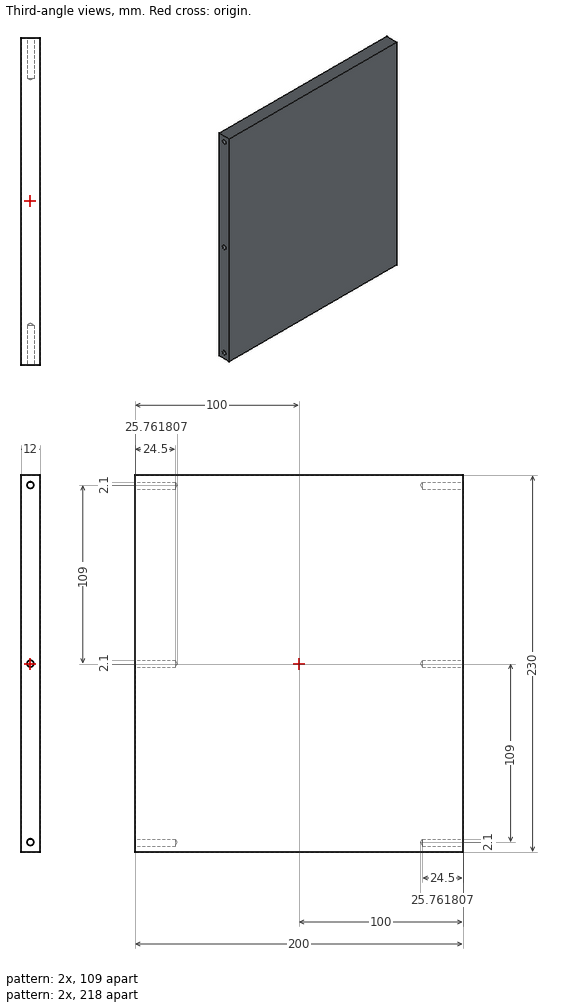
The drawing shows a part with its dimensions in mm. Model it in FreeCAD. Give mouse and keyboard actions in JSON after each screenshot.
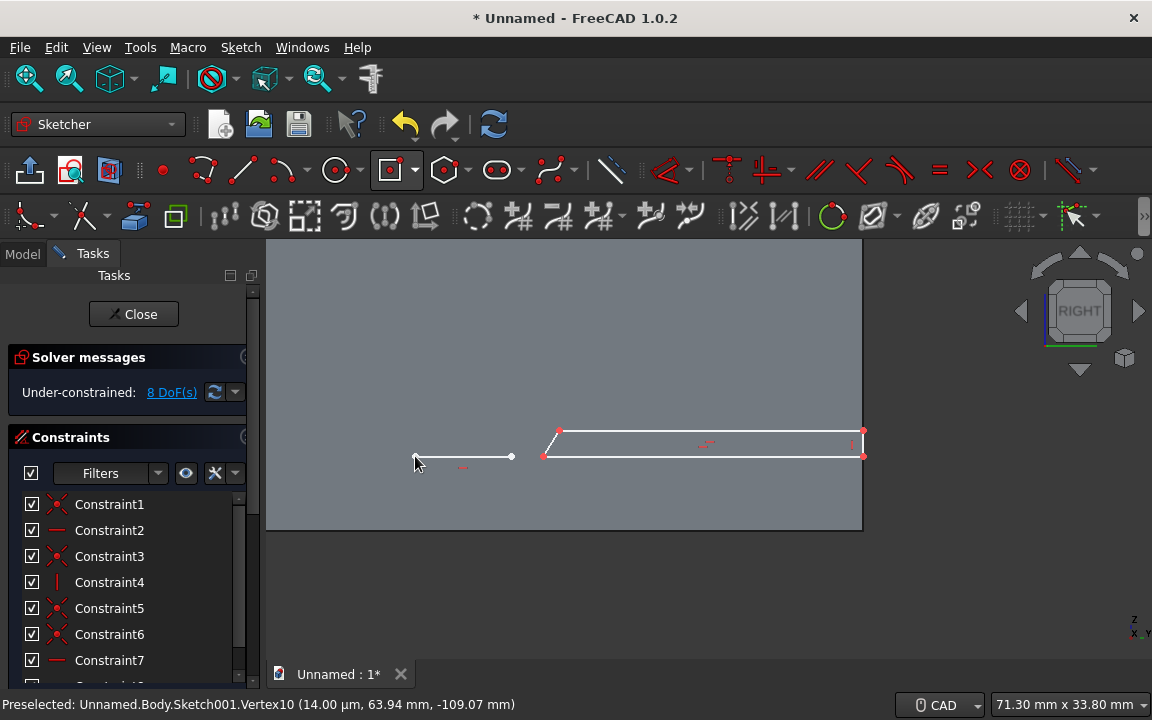
{"action": "left_click", "coordinate": [482, 457]}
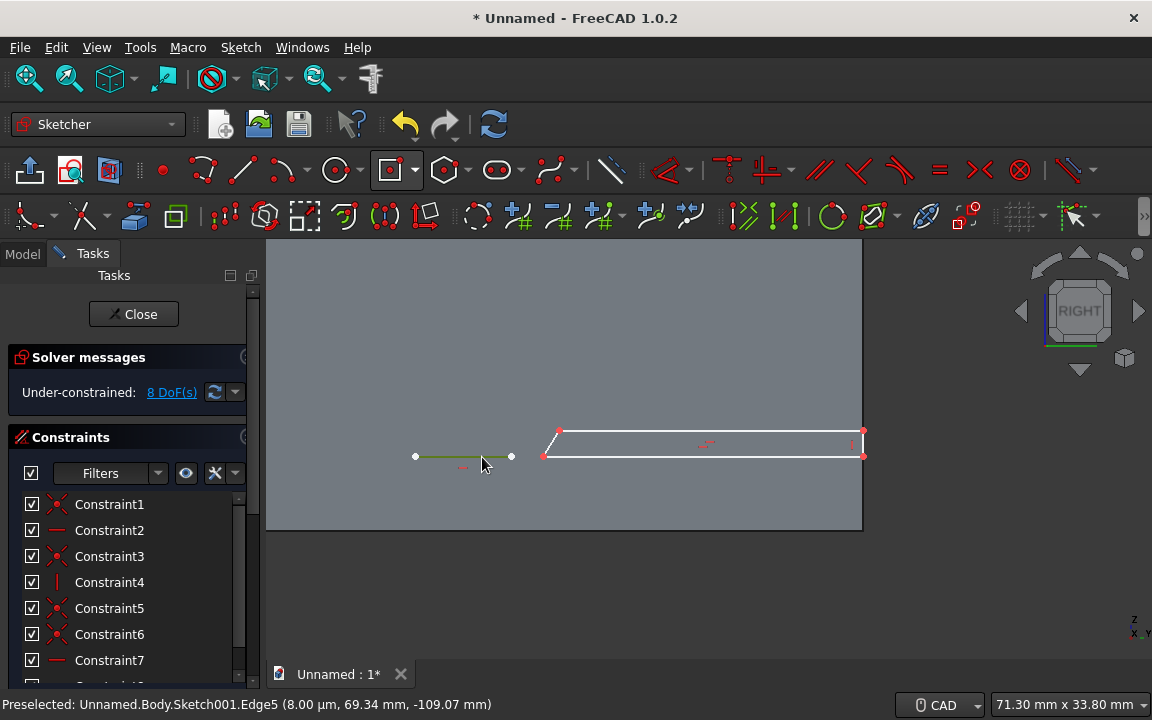
{"action": "left_click", "coordinate": [612, 170]}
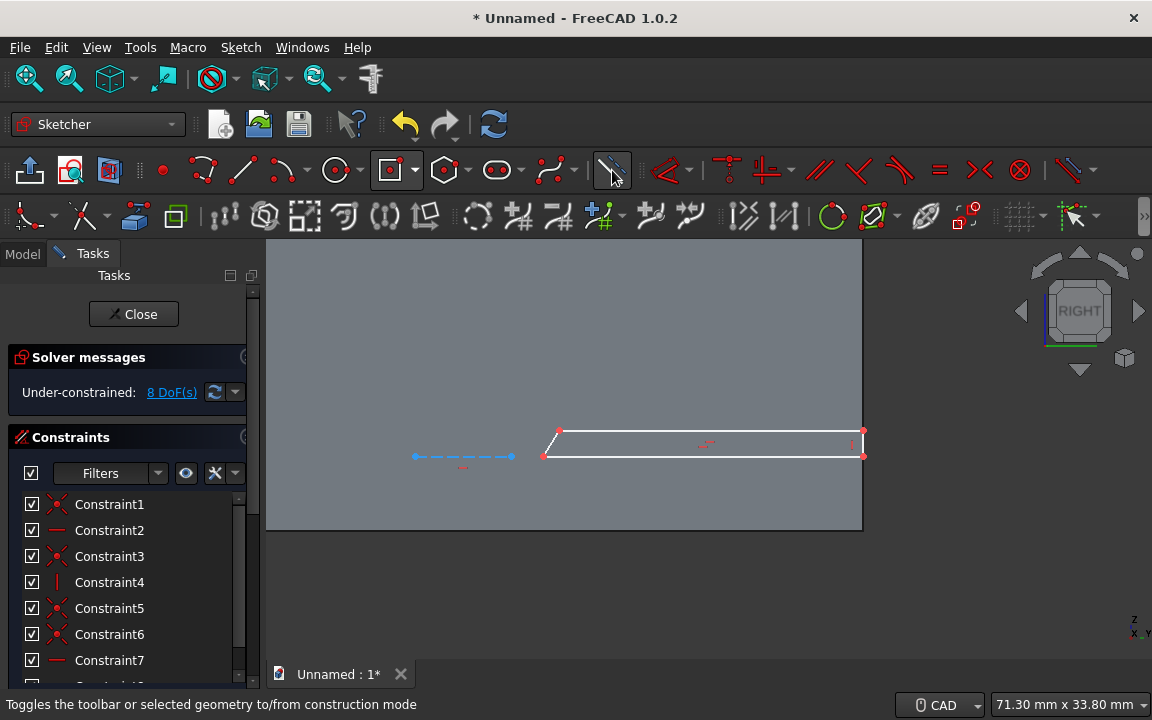
{"action": "left_click", "coordinate": [666, 170]}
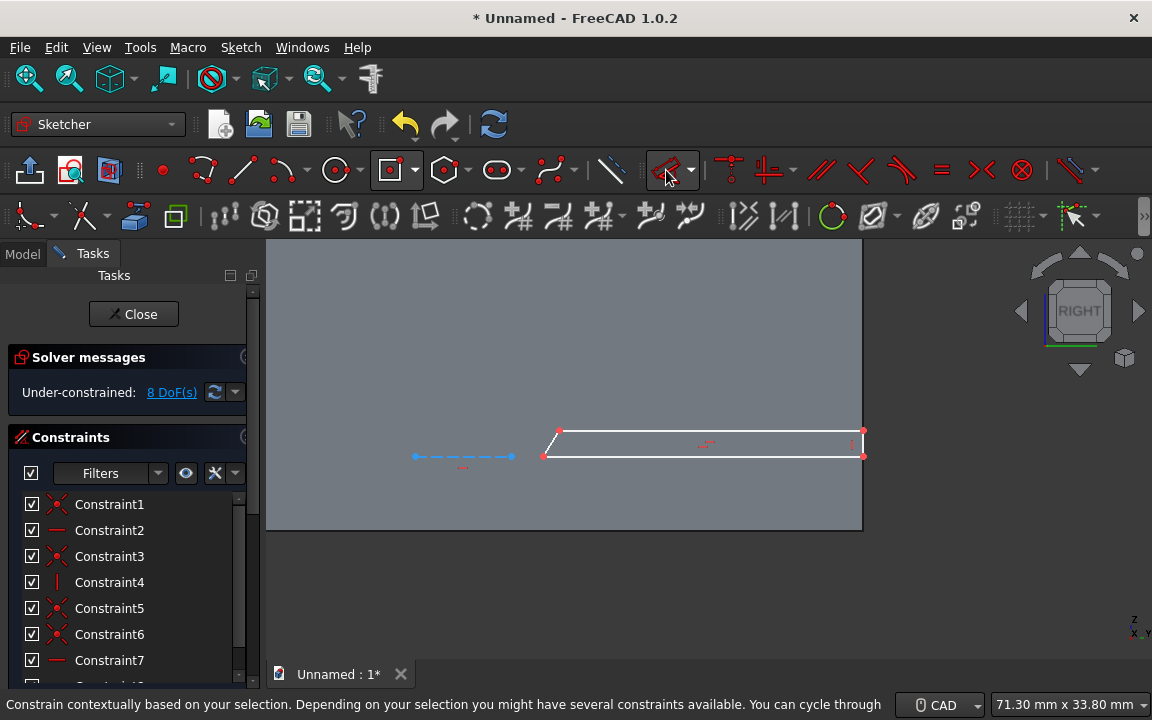
{"action": "scroll", "coordinate": [863, 447], "scroll_direction": "up", "scroll_amount": 3}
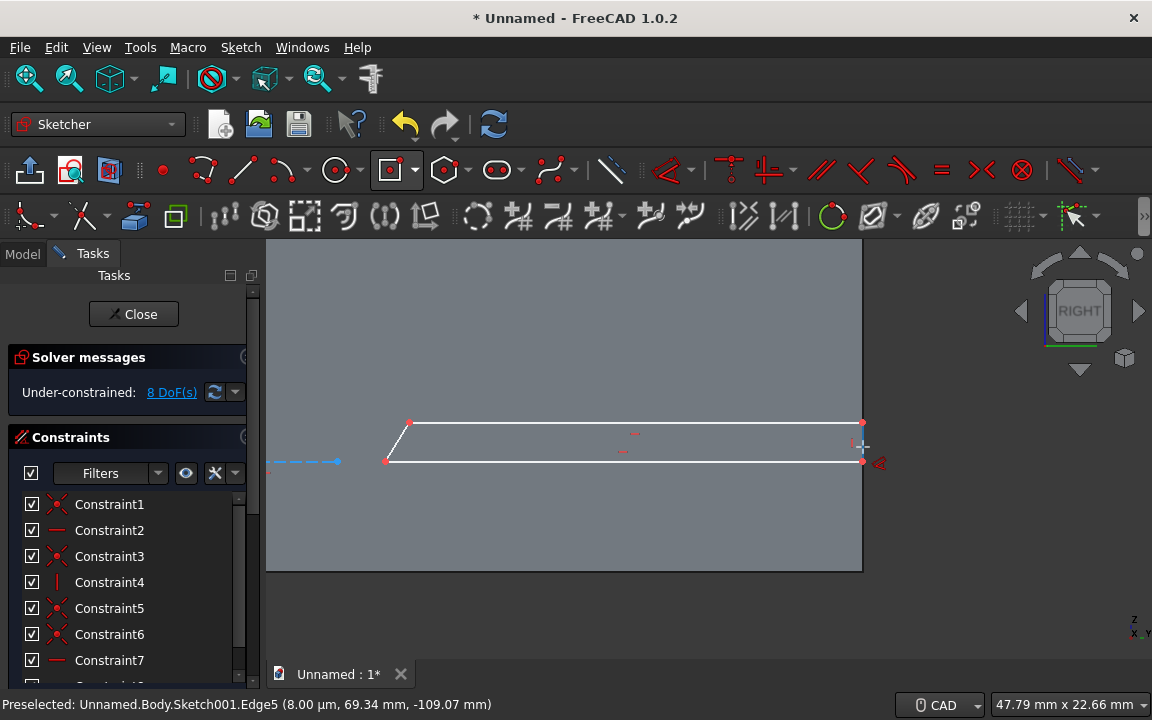
{"action": "left_click", "coordinate": [862, 446]}
{"action": "left_click", "coordinate": [896, 441]}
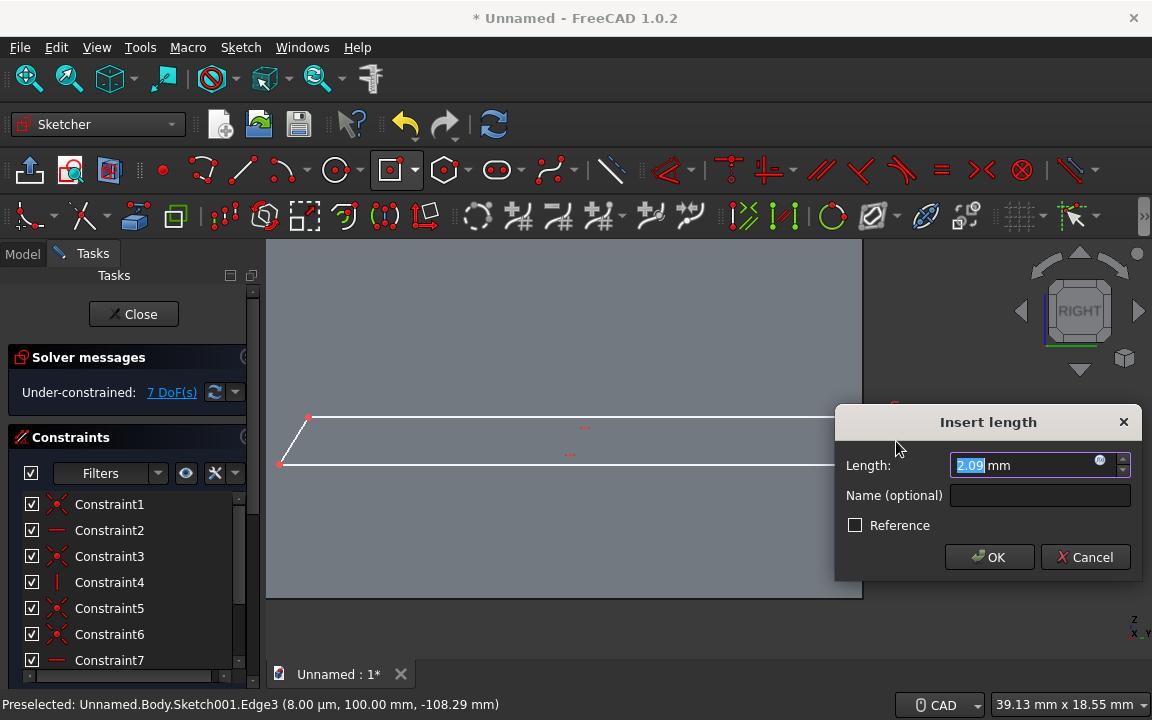
{"action": "type", "text": "2.1"}
{"action": "key", "text": "Return"}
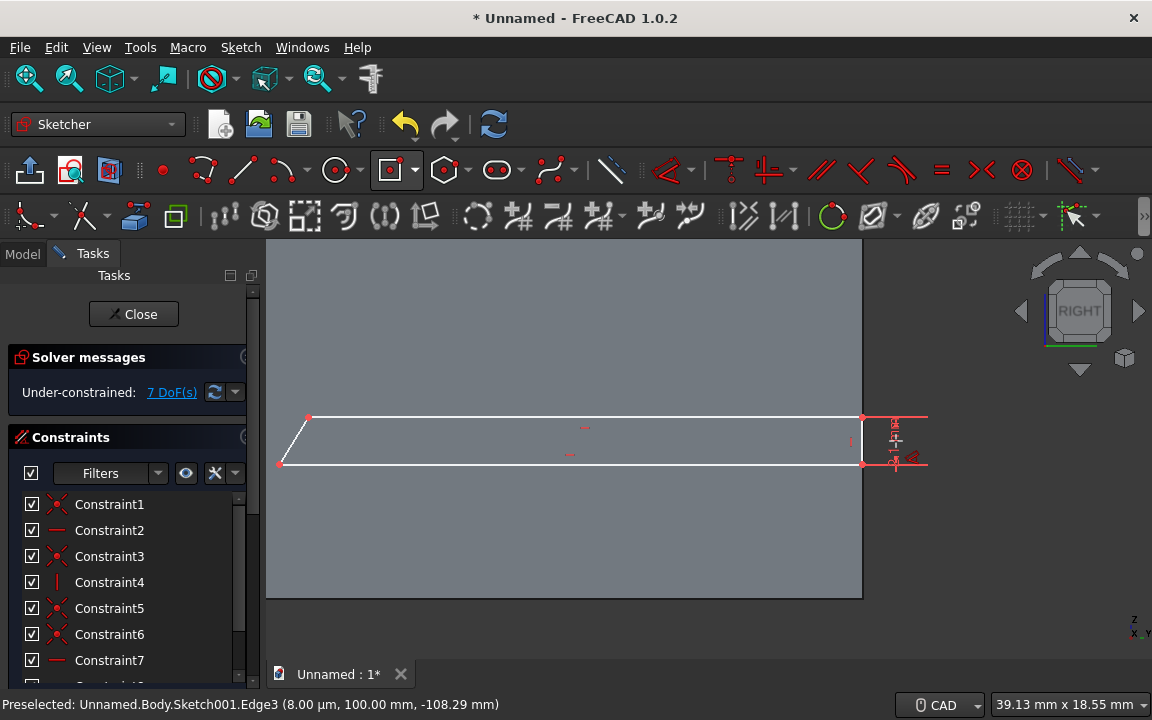
{"action": "left_click", "coordinate": [696, 417]}
{"action": "left_click", "coordinate": [585, 383]}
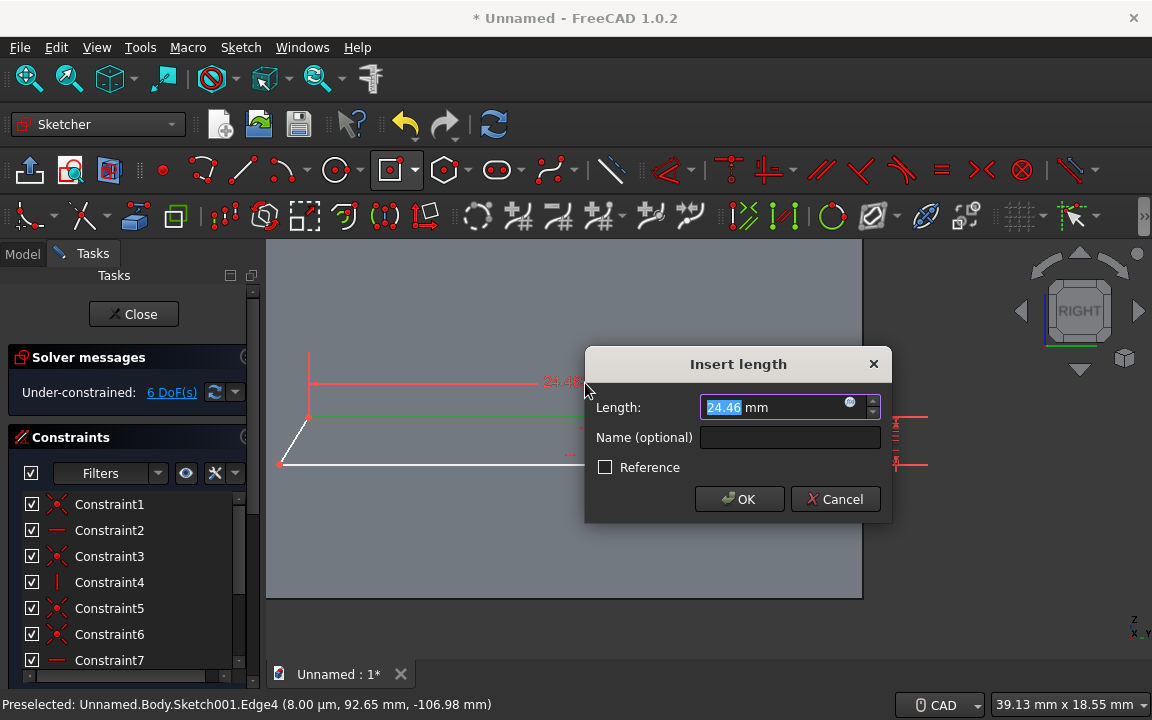
{"action": "type", "text": "24.5"}
{"action": "key", "text": "Return"}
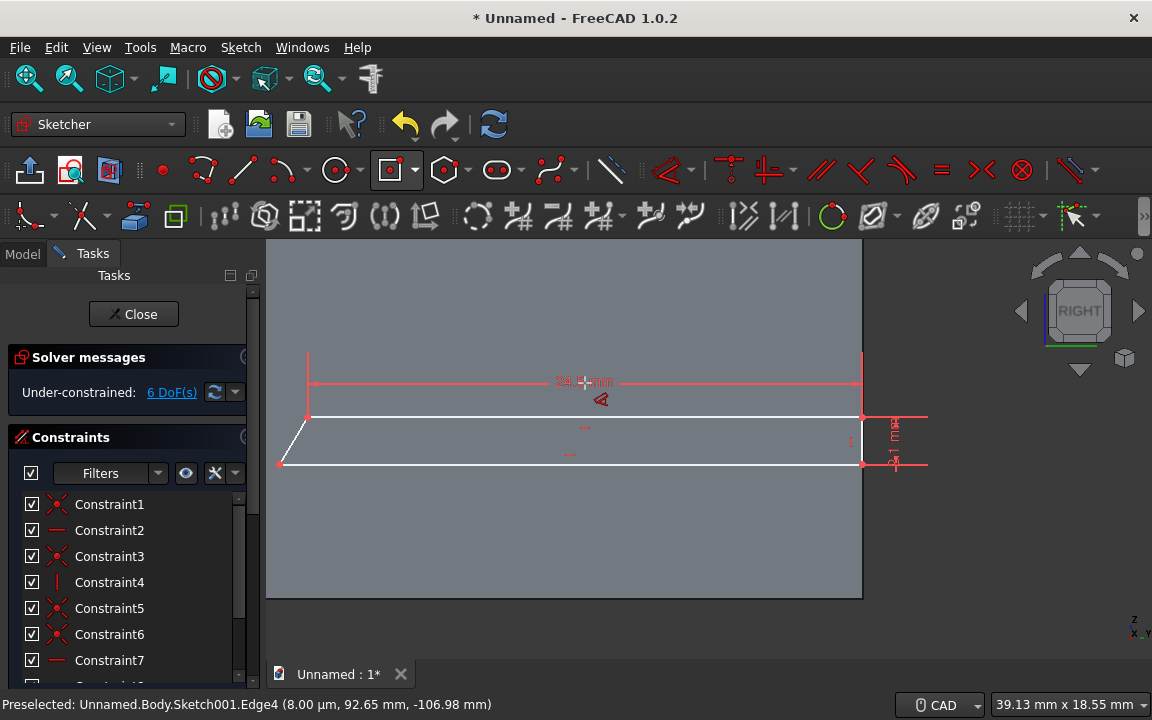
{"action": "scroll", "coordinate": [867, 461], "scroll_direction": "down", "scroll_amount": 3}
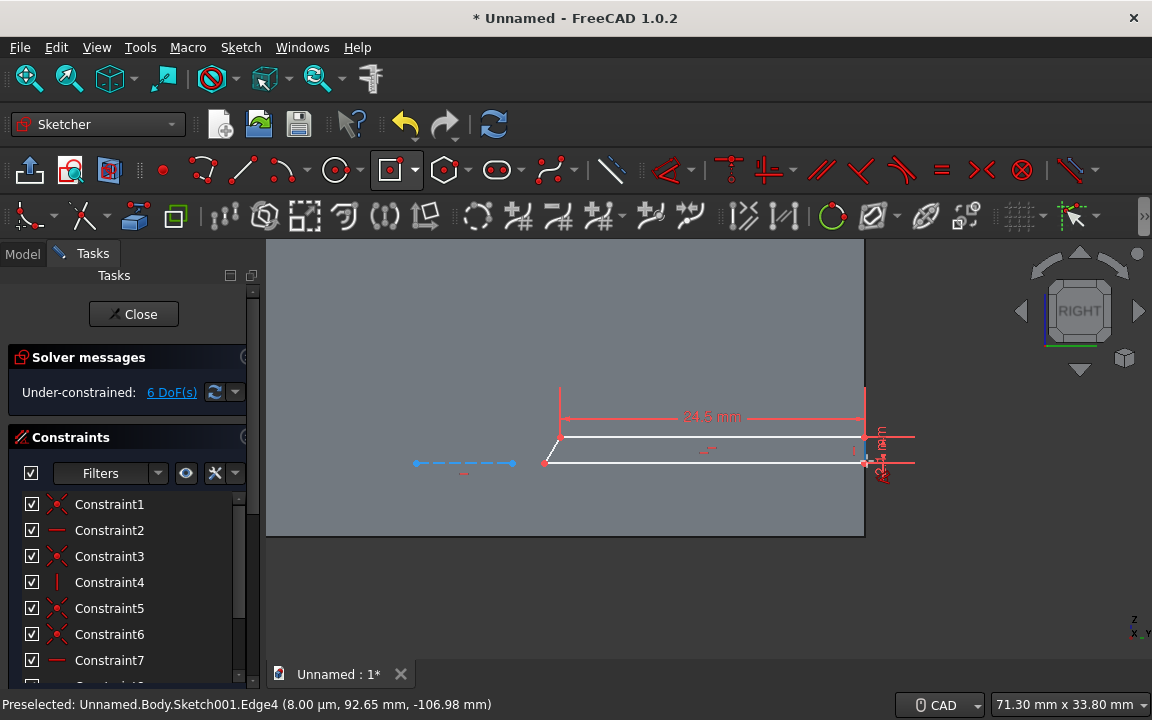
{"action": "left_click", "coordinate": [545, 463]}
{"action": "left_click", "coordinate": [579, 365]}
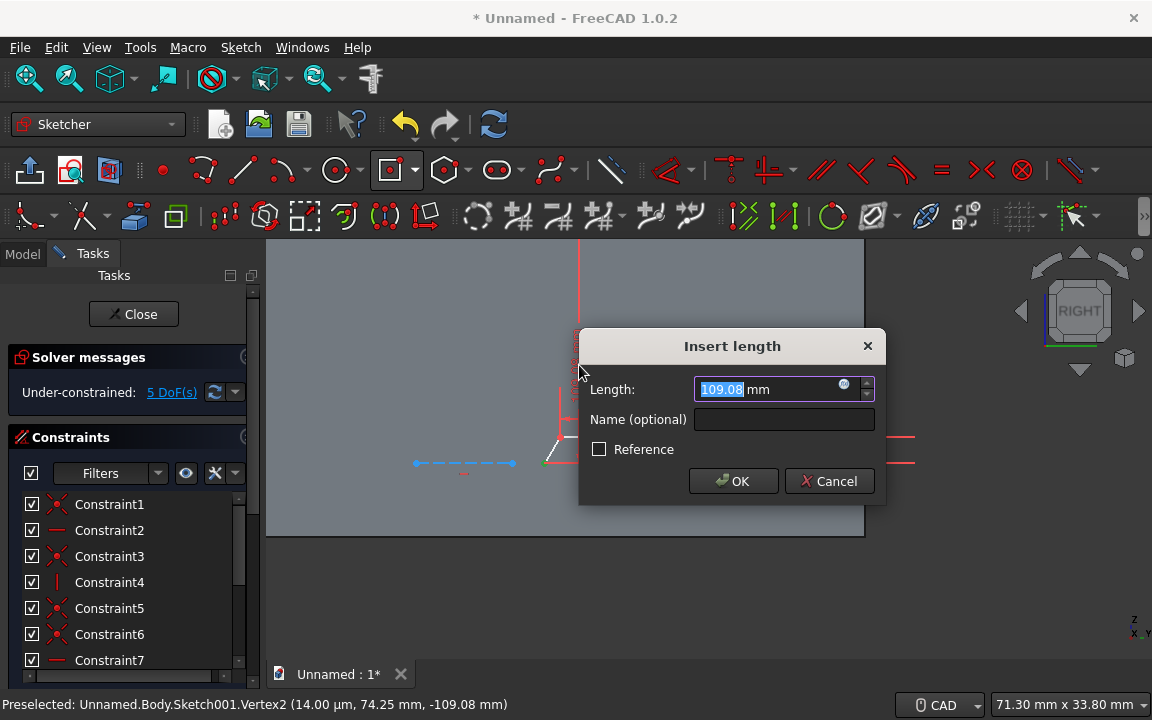
{"action": "type", "text": "109"}
{"action": "key", "text": "Return"}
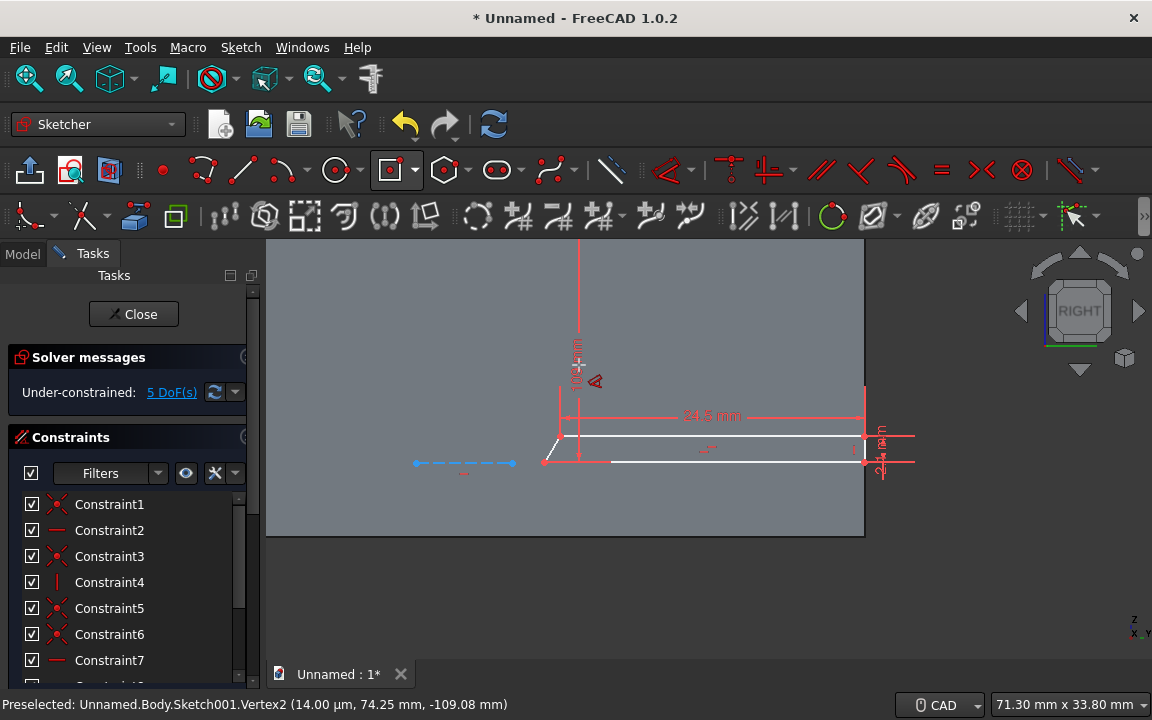
{"action": "left_click", "coordinate": [865, 462]}
{"action": "left_click", "coordinate": [579, 496]}